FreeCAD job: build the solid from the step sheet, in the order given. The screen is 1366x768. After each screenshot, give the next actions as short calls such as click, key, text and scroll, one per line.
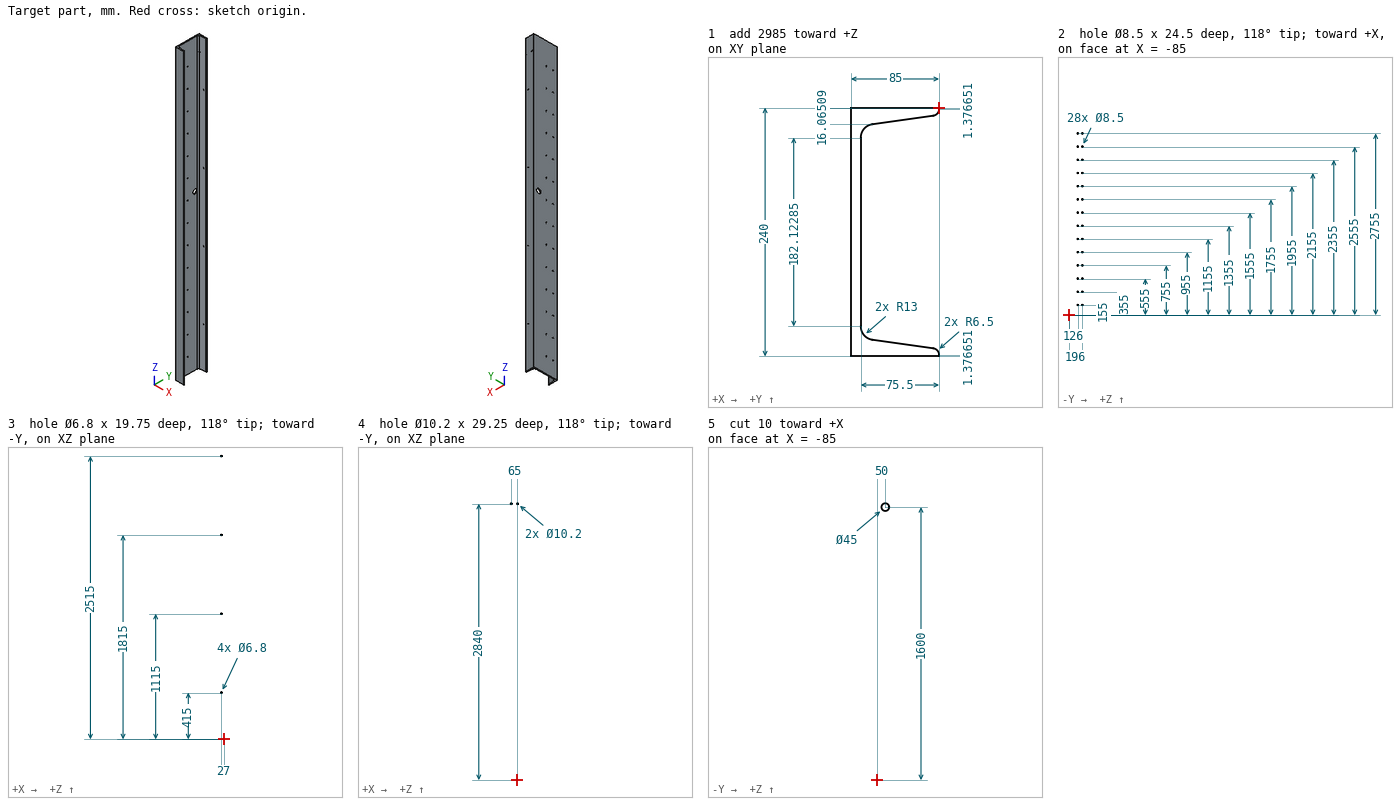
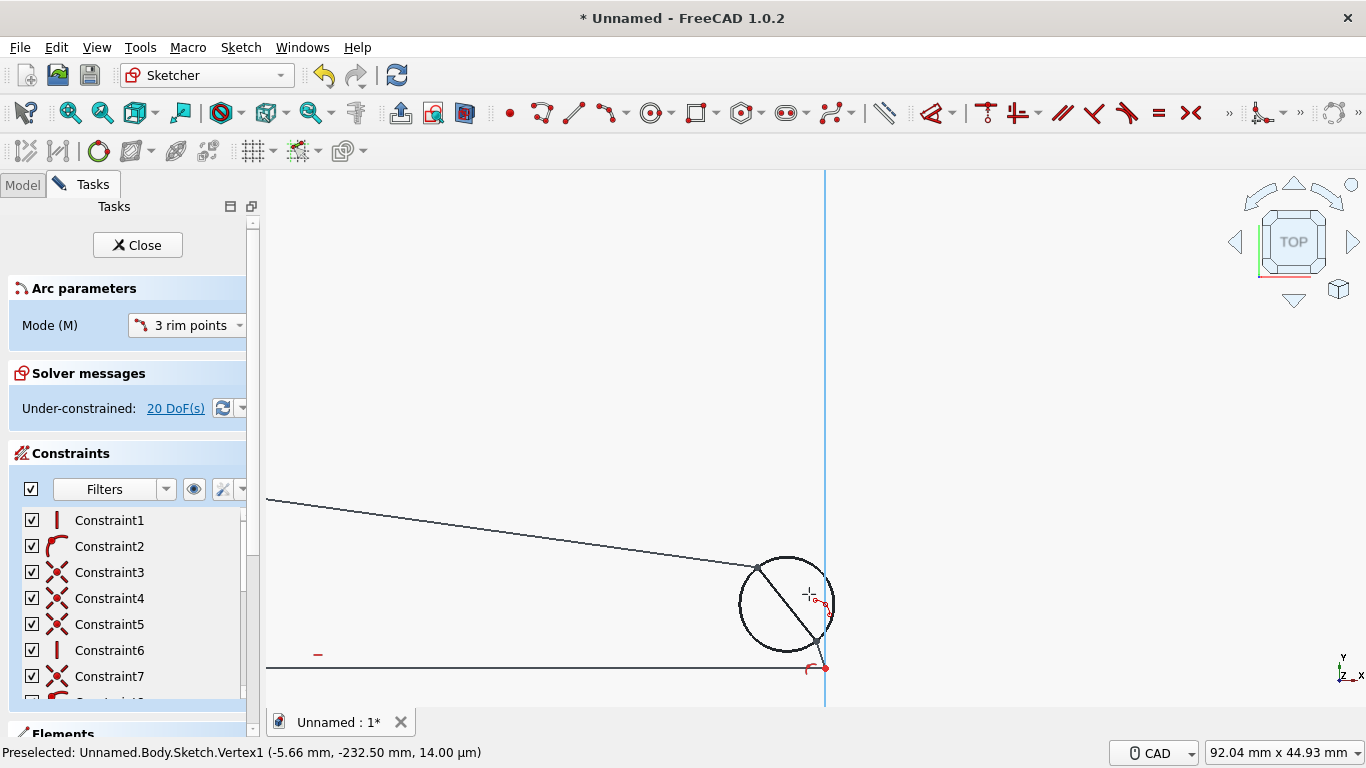
click(806, 590)
key(Escape)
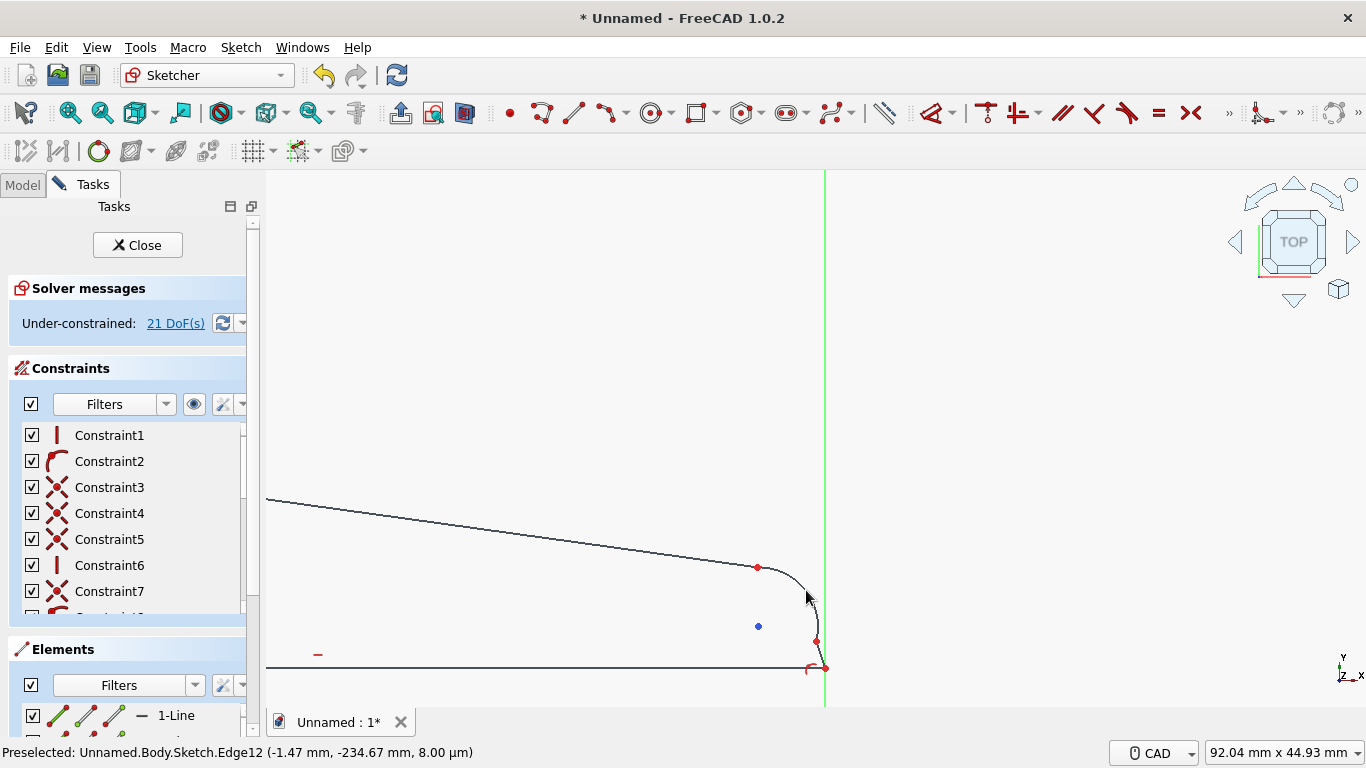
scroll(801, 590, down, 11)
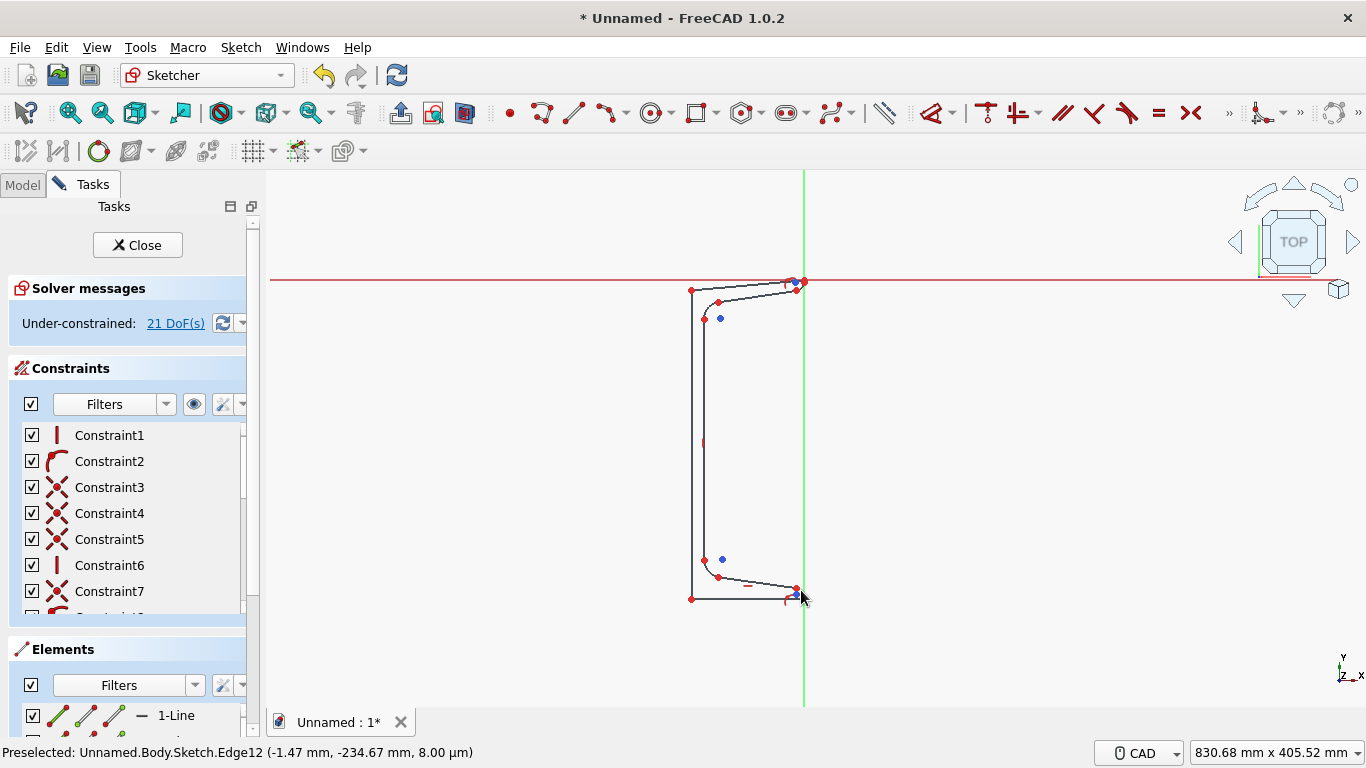
click(773, 585)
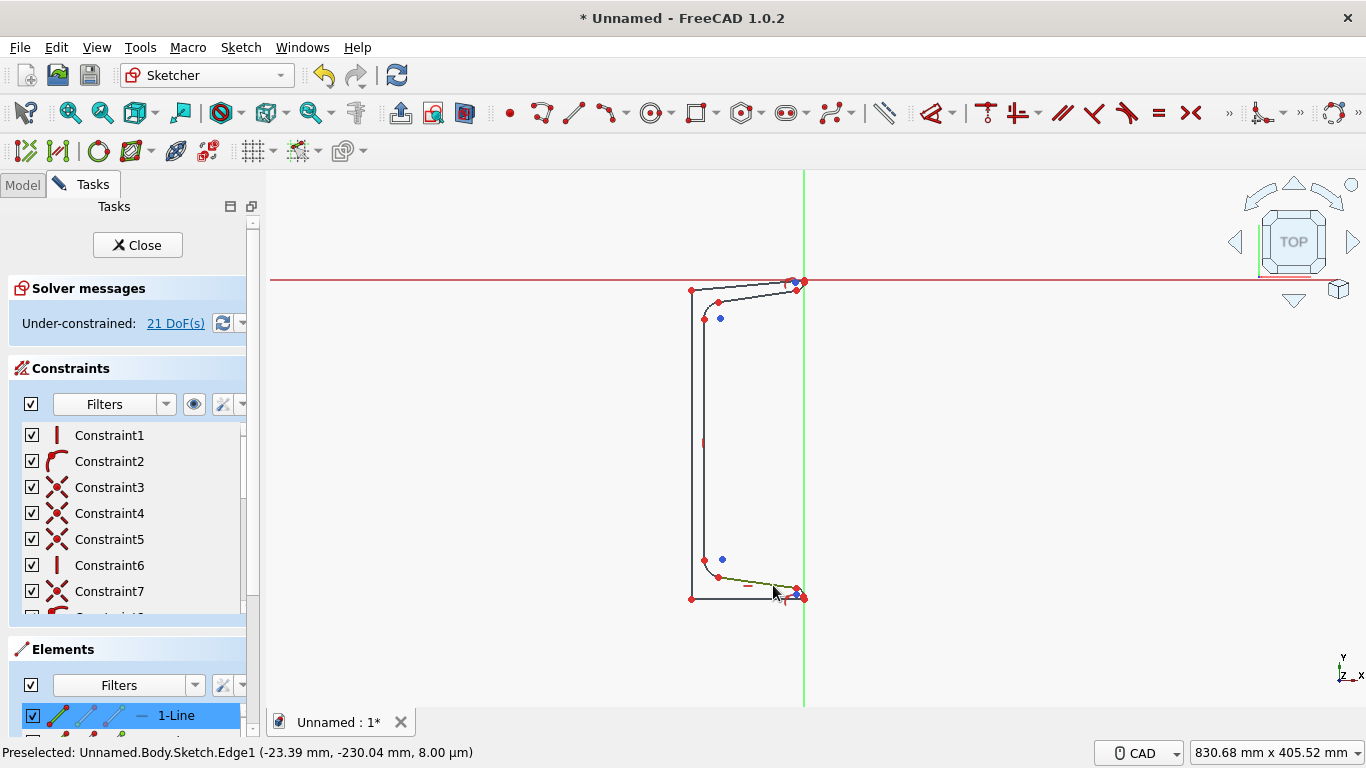
click(709, 571)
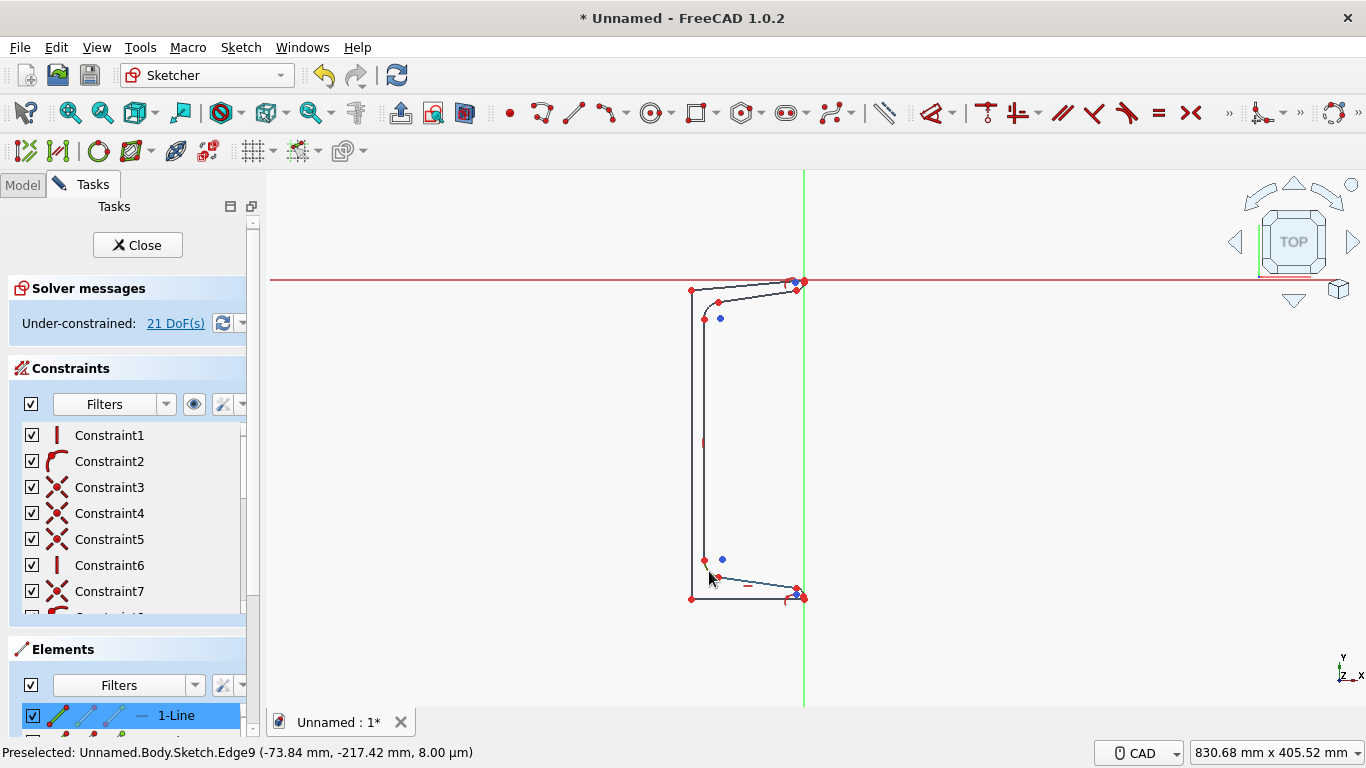
click(1128, 114)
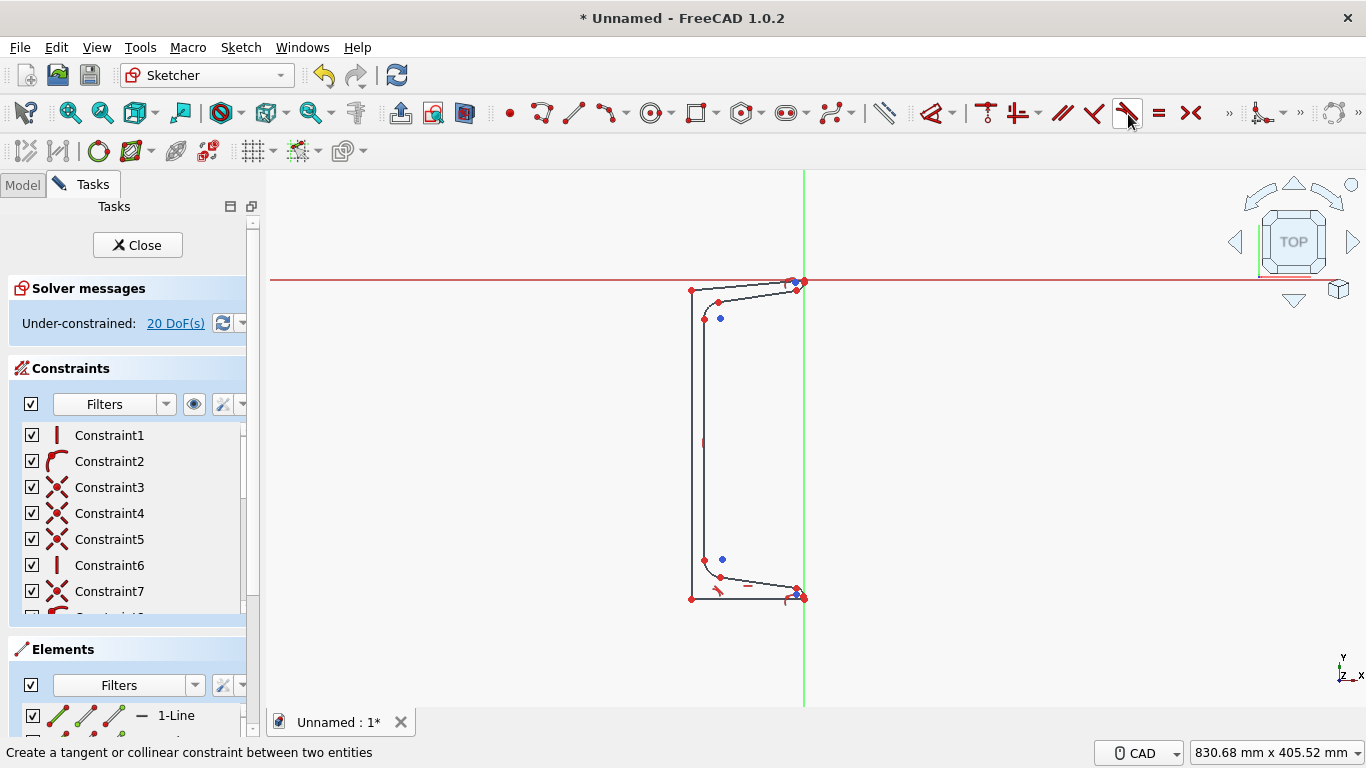
click(774, 585)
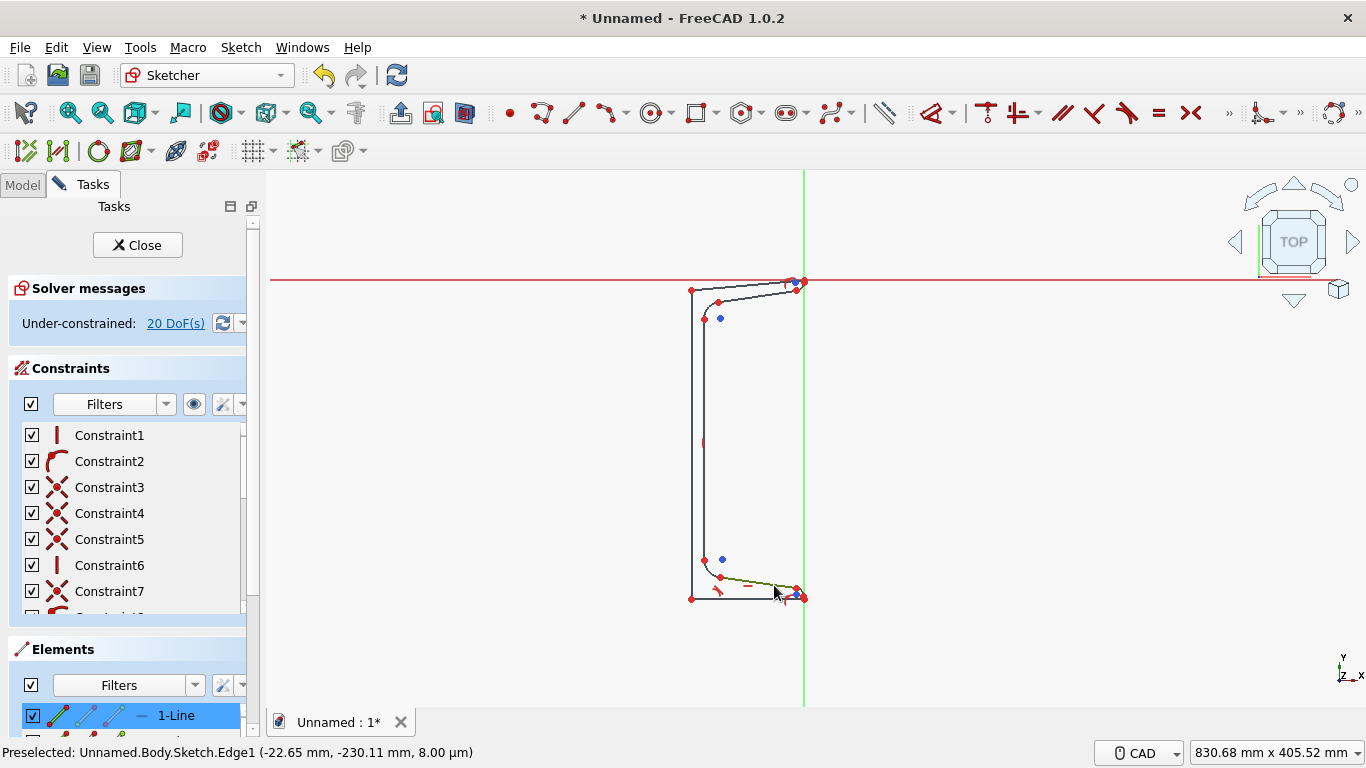
scroll(802, 591, up, 5)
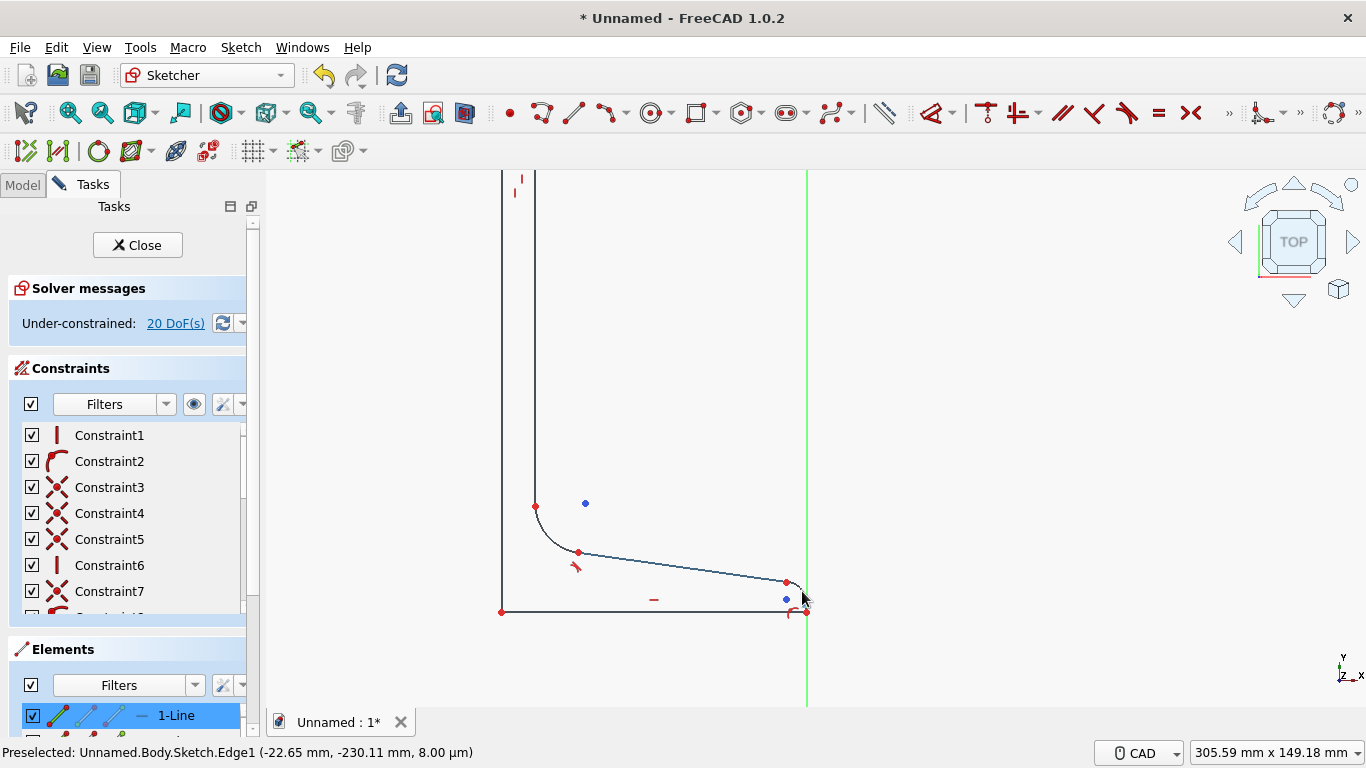
click(801, 589)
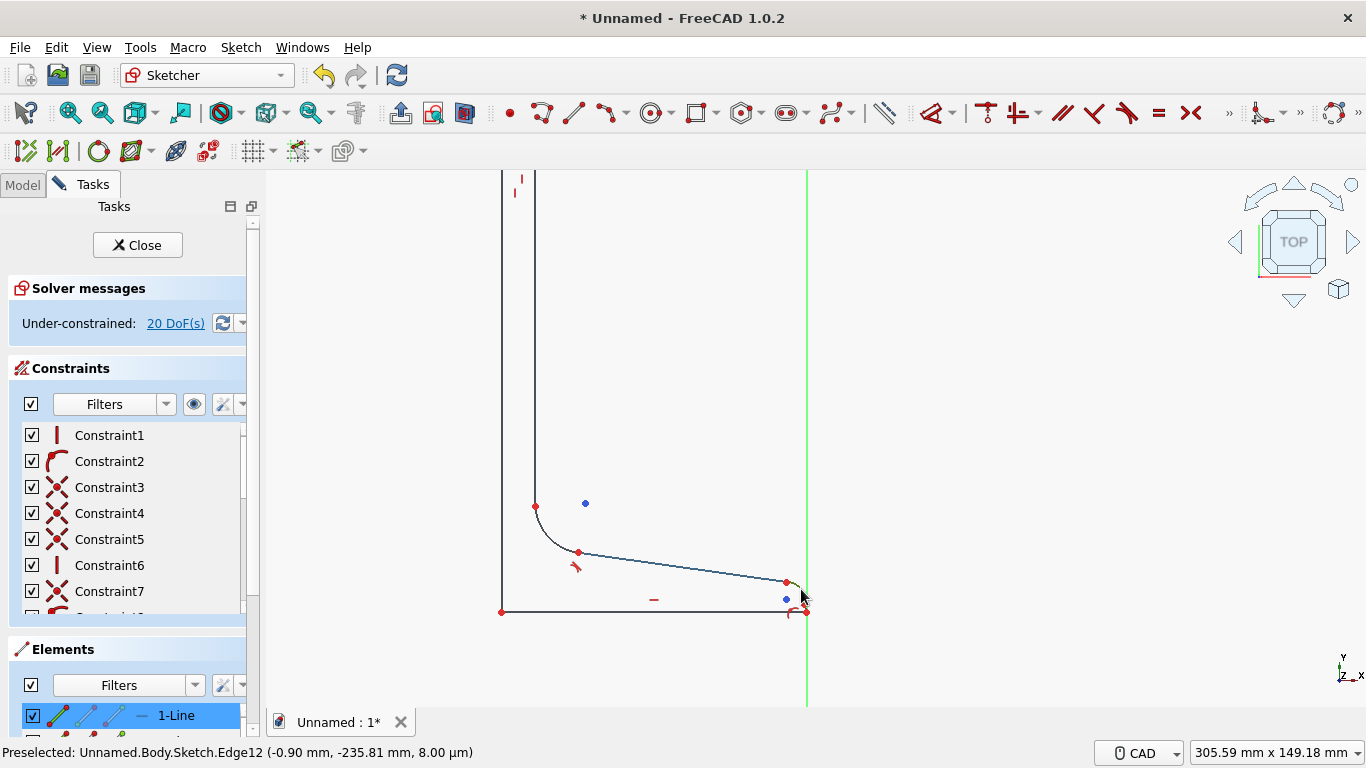
click(1128, 114)